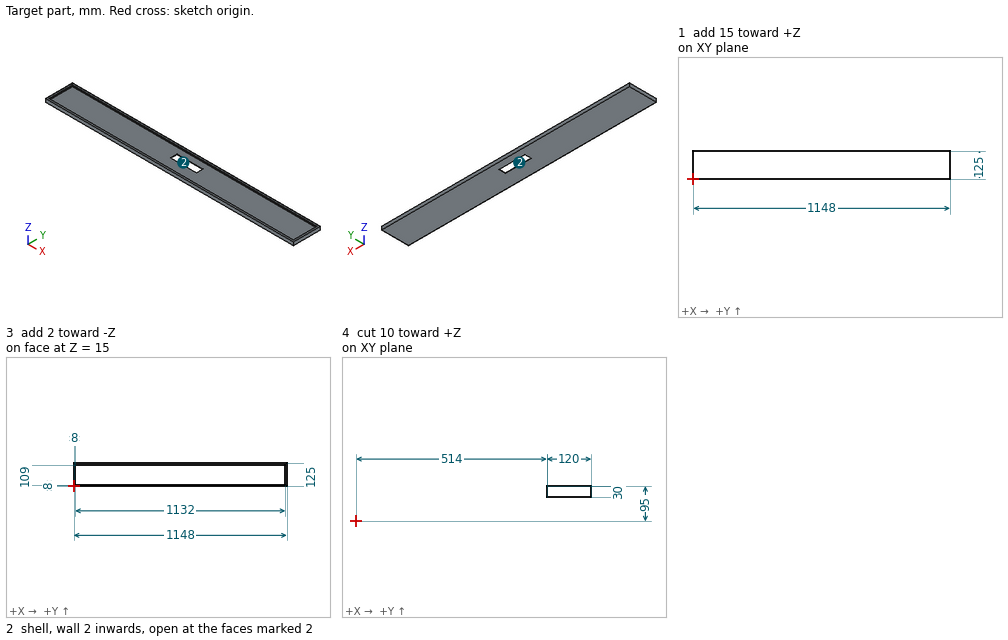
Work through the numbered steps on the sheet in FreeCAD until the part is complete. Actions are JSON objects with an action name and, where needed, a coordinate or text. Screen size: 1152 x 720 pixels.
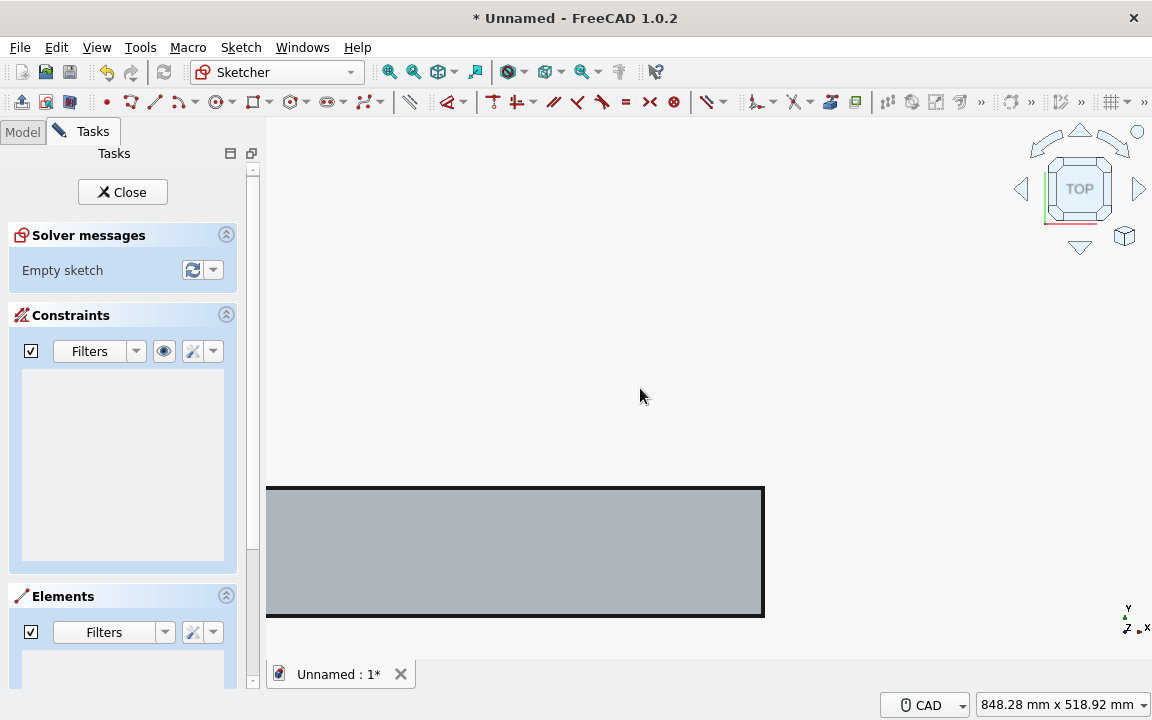
{"action": "scroll", "coordinate": [987, 254], "scroll_direction": "down", "scroll_amount": 4}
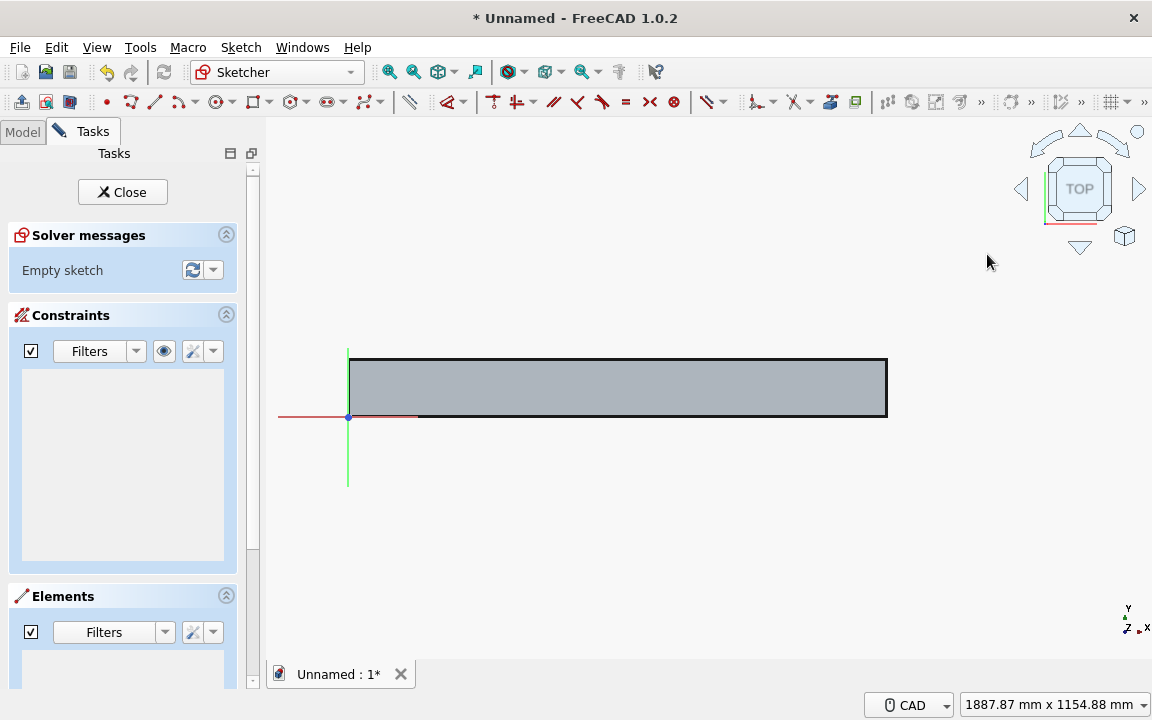
{"action": "left_click", "coordinate": [254, 102]}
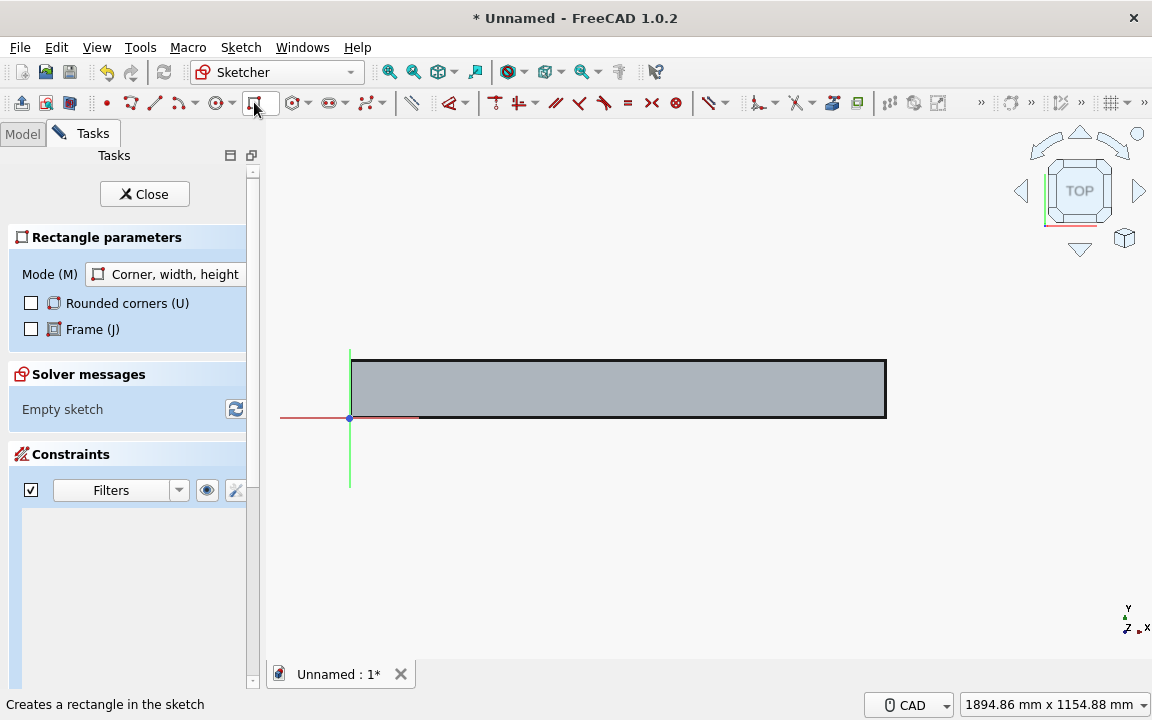
{"action": "left_click", "coordinate": [350, 418]}
{"action": "mouse_move", "coordinate": [886, 360]}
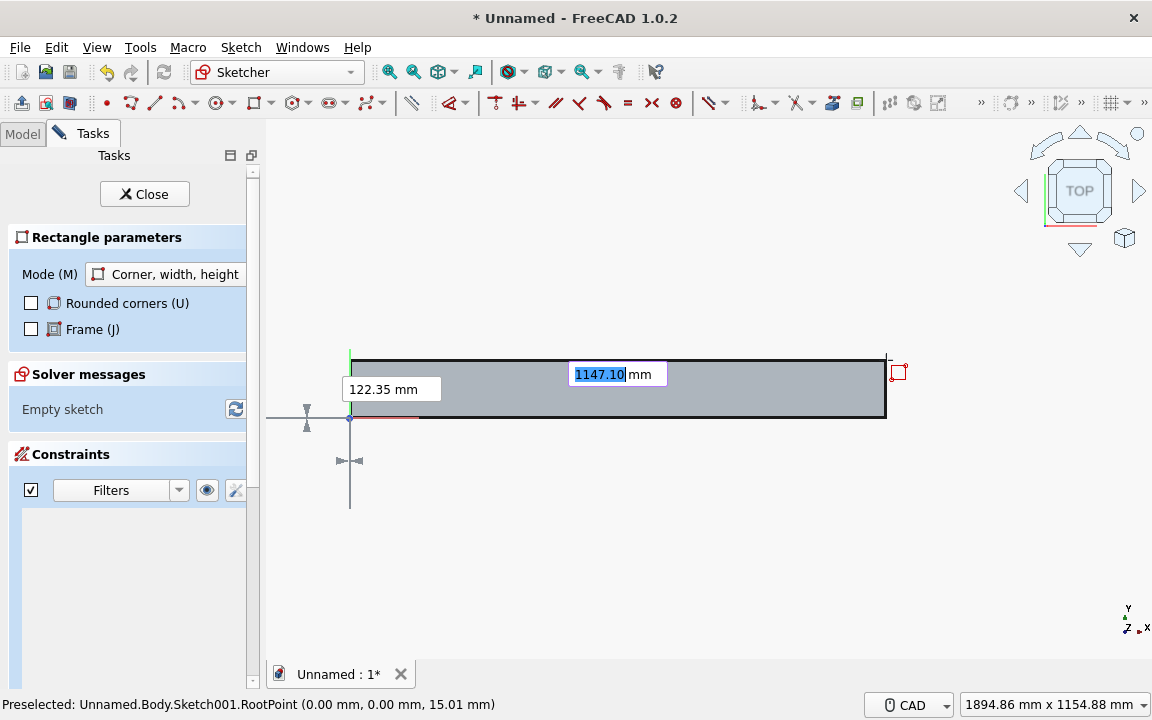
{"action": "type", "text": "1148"}
{"action": "key", "text": "Tab"}
{"action": "type", "text": "125"}
{"action": "key", "text": "Return"}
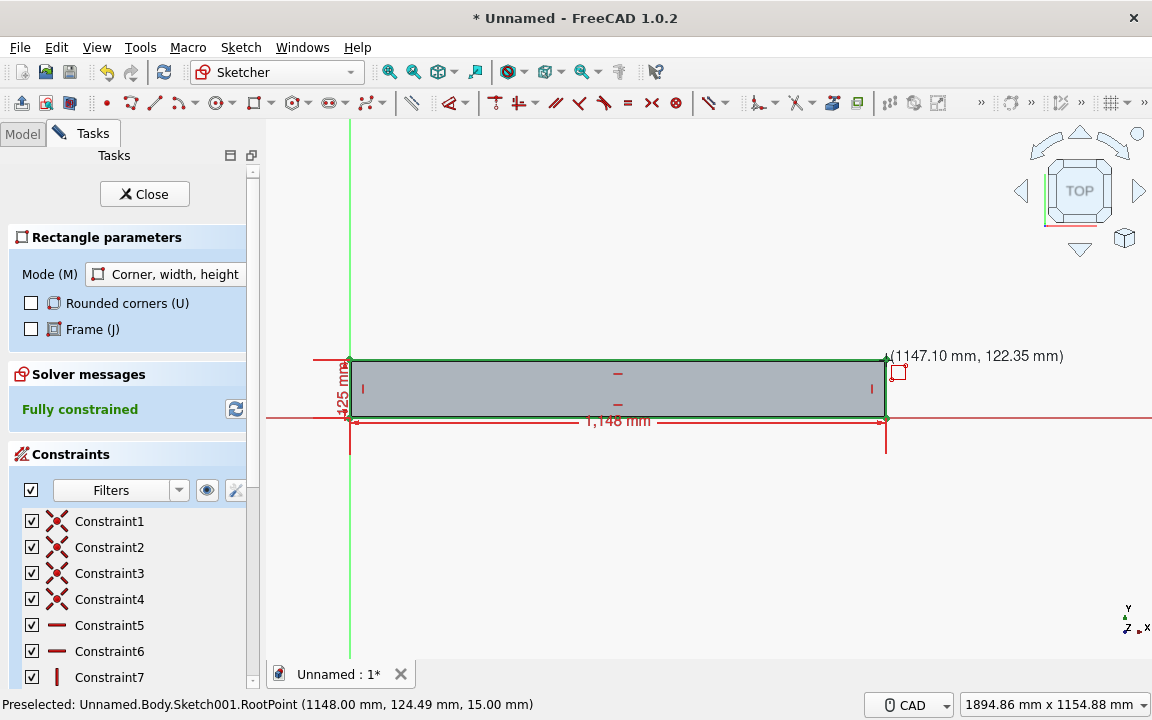
{"action": "scroll", "coordinate": [353, 364], "scroll_direction": "up", "scroll_amount": 8}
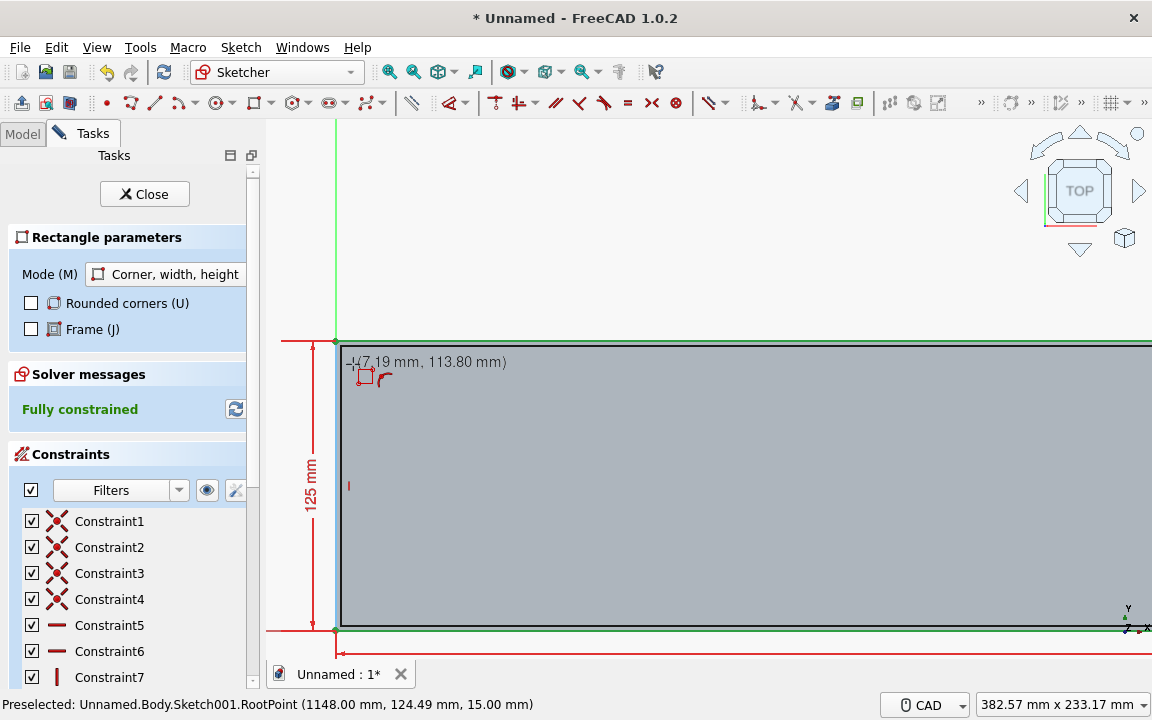
{"action": "left_click", "coordinate": [354, 360]}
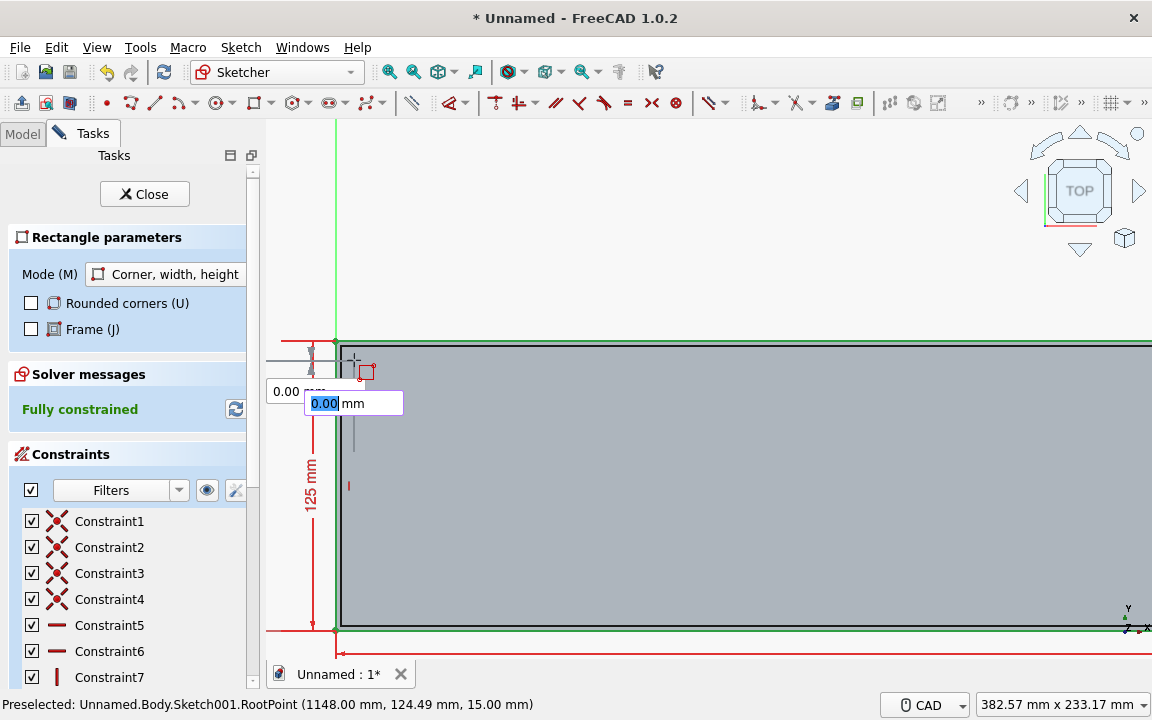
{"action": "scroll", "coordinate": [381, 364], "scroll_direction": "down", "scroll_amount": 8}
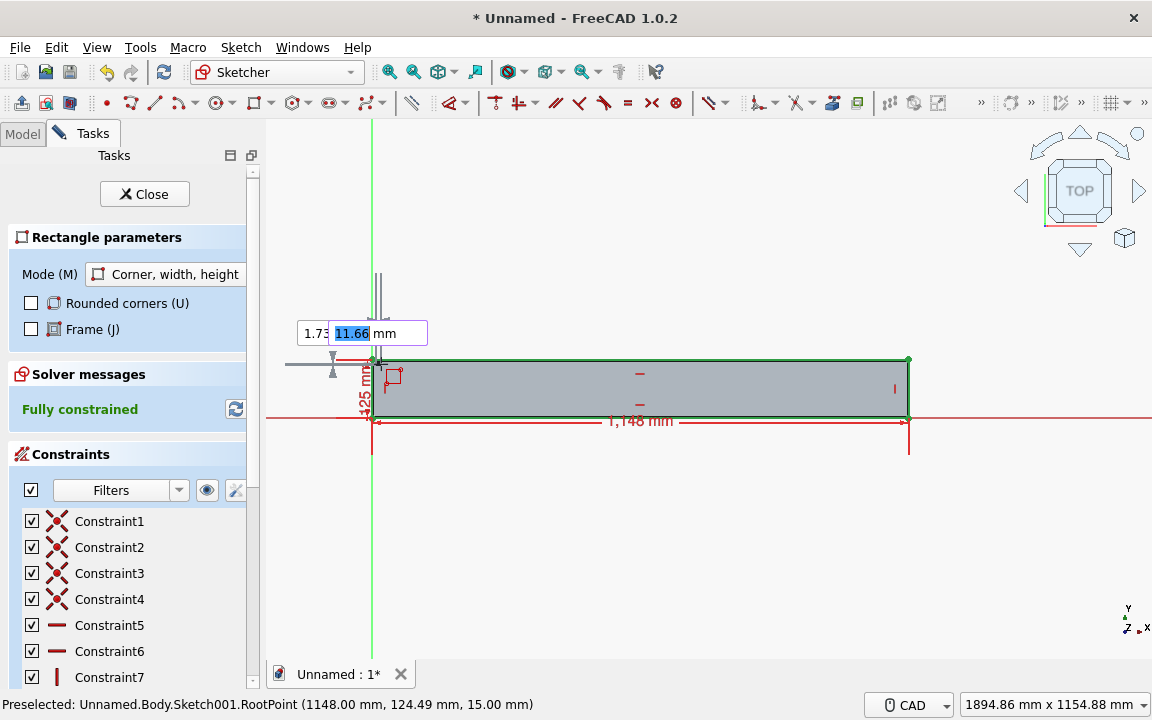
{"action": "scroll", "coordinate": [905, 414], "scroll_direction": "up", "scroll_amount": 8}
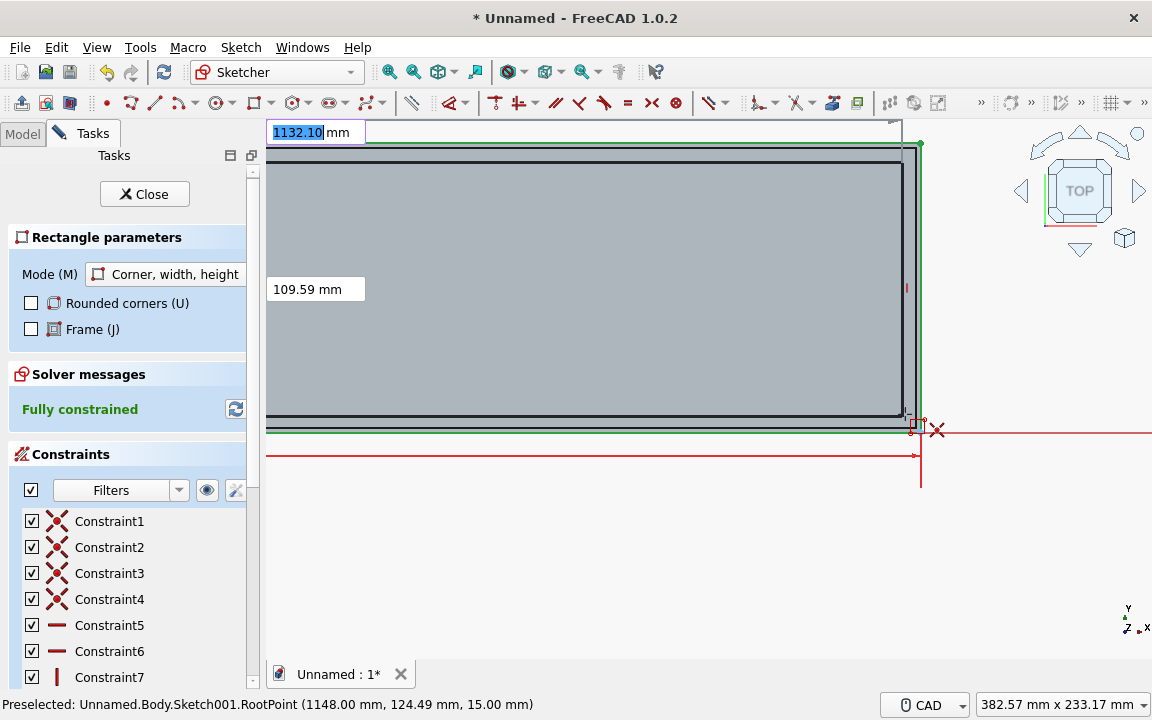
{"action": "left_click", "coordinate": [902, 414]}
{"action": "key", "text": "Escape"}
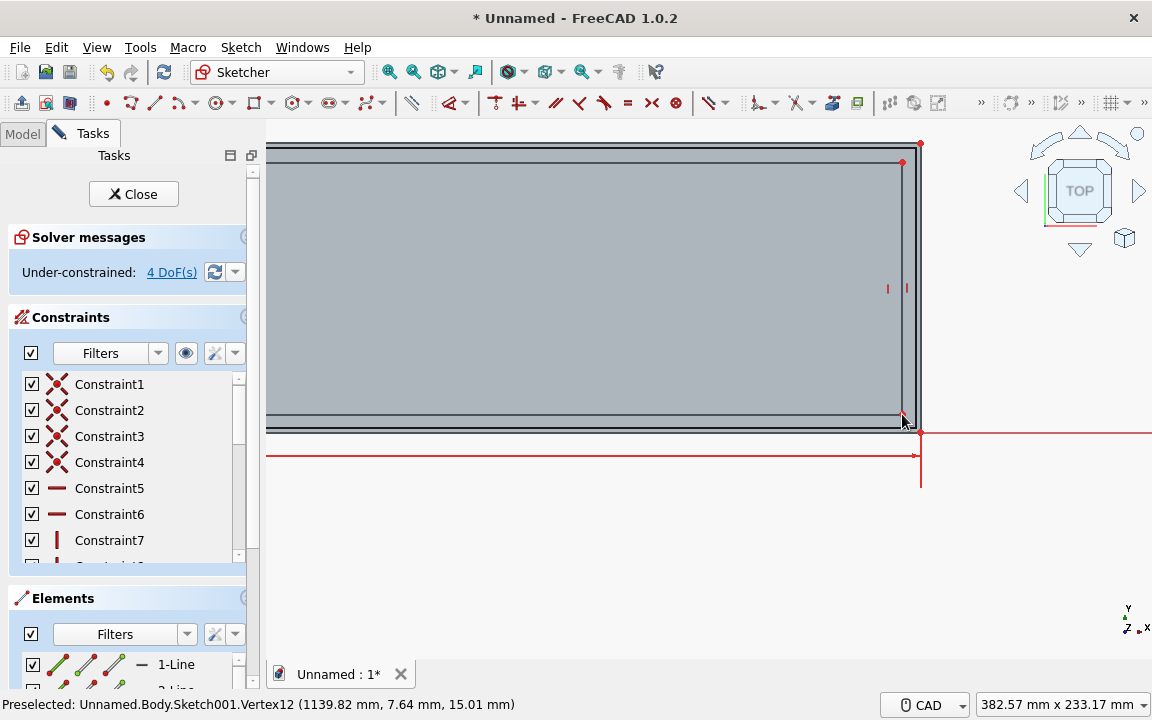
{"action": "left_click", "coordinate": [450, 104]}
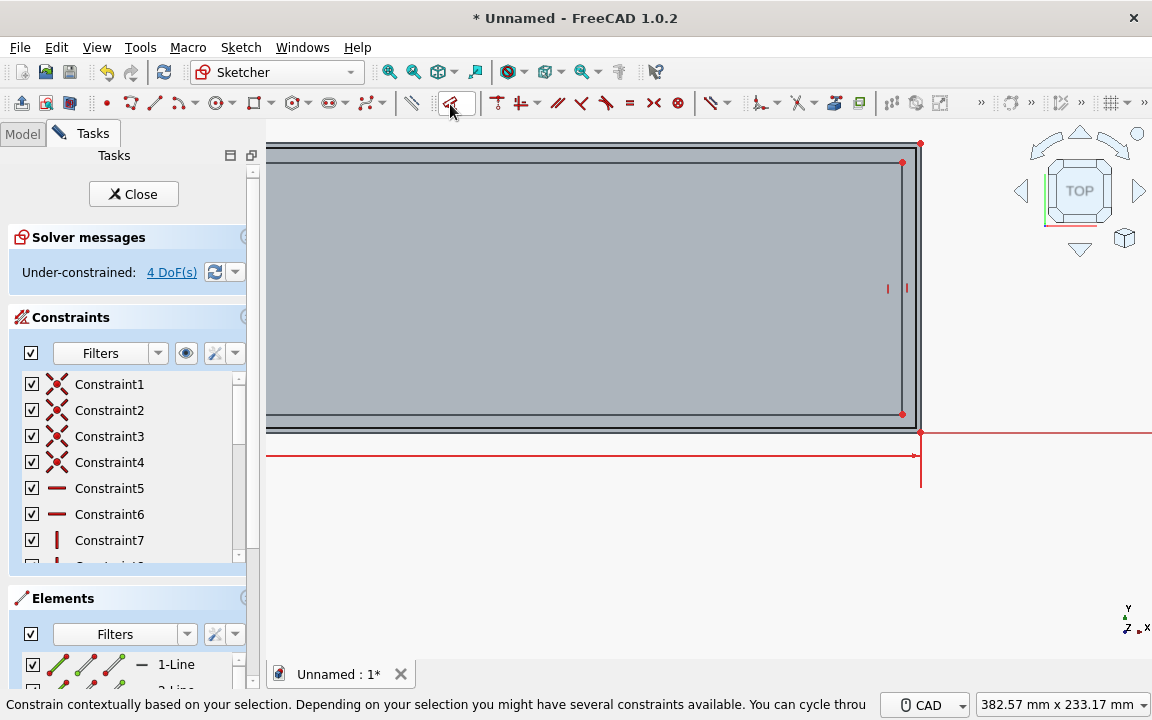
{"action": "scroll", "coordinate": [906, 415], "scroll_direction": "down", "scroll_amount": 8}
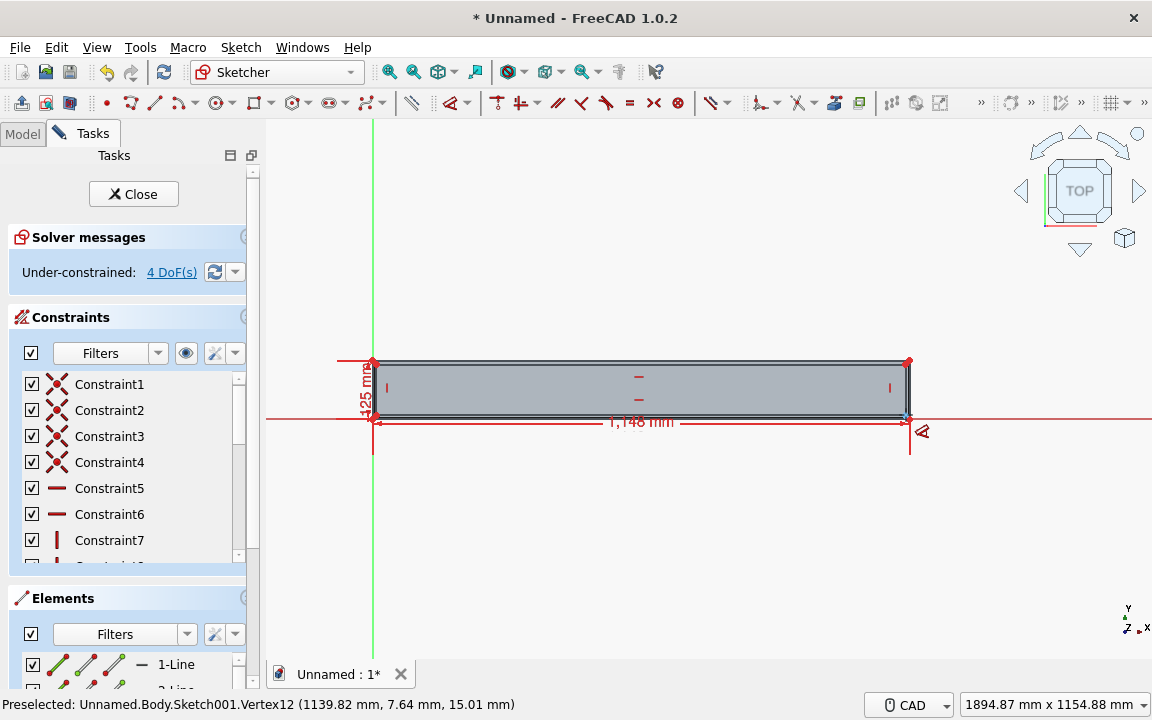
{"action": "scroll", "coordinate": [376, 365], "scroll_direction": "up", "scroll_amount": 12}